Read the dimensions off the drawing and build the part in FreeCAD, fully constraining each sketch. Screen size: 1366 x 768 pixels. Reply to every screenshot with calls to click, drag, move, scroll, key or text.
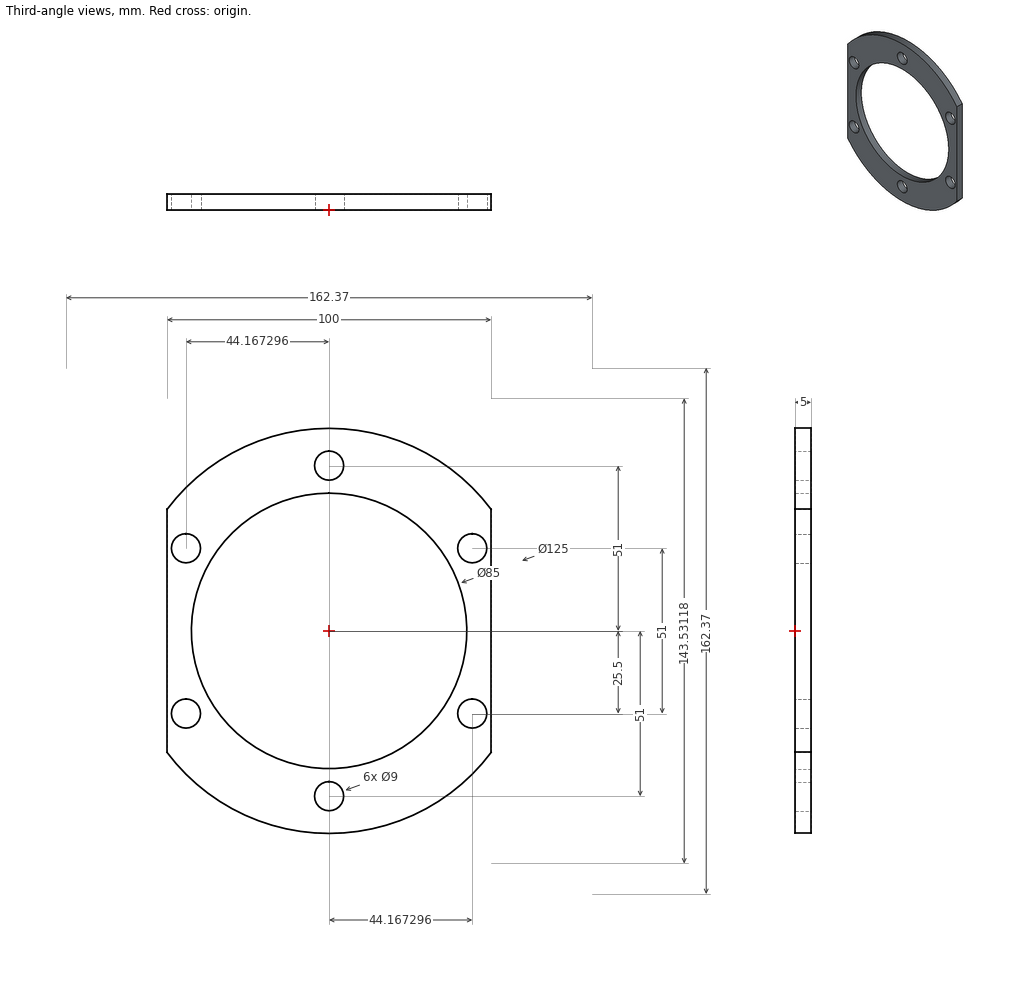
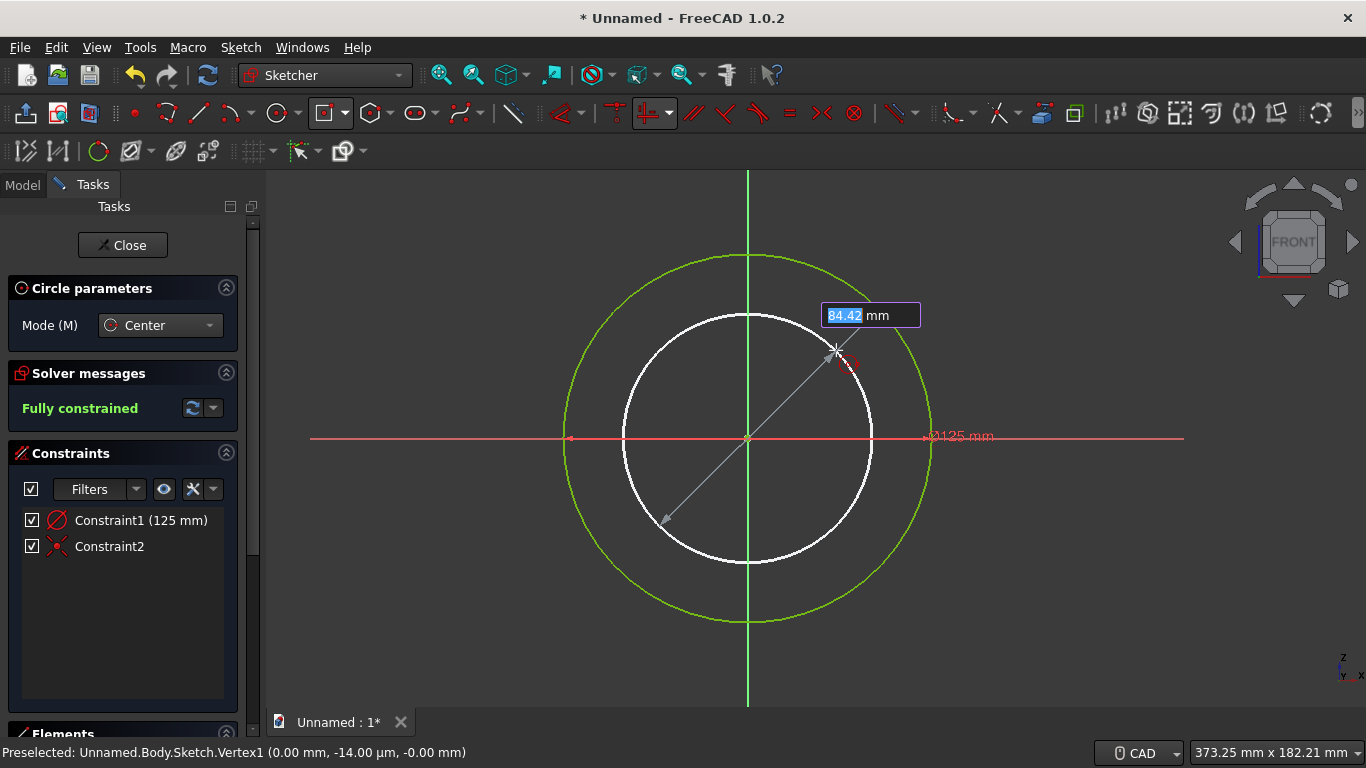
text(85)
key(Return)
key(Escape)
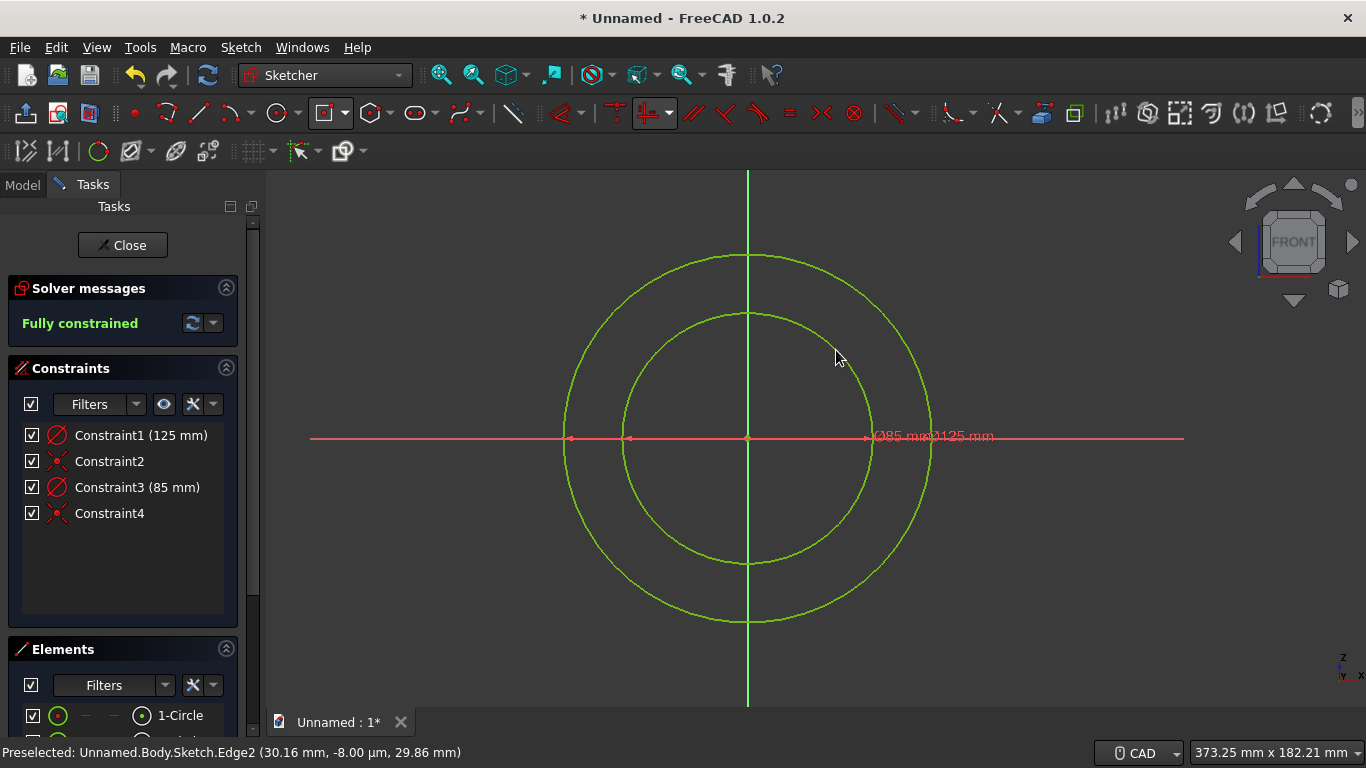
click(123, 245)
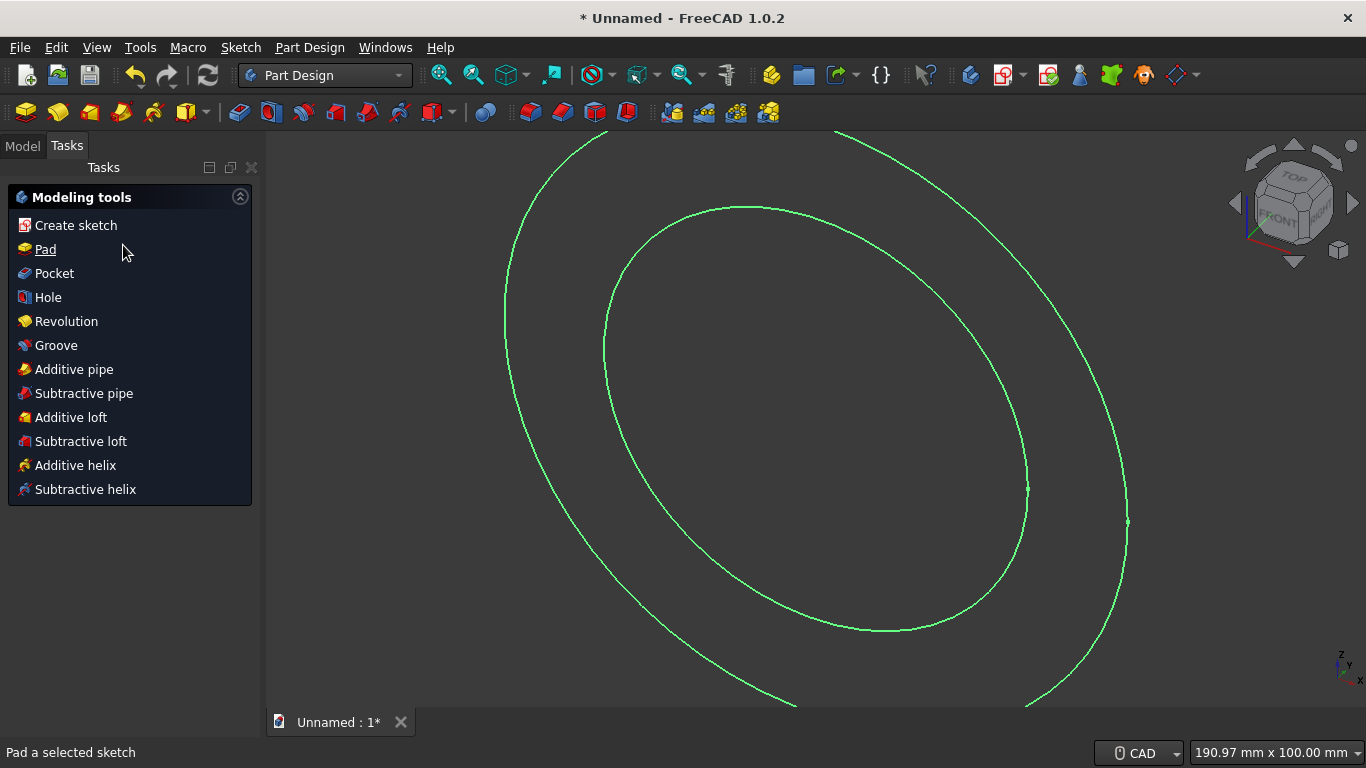
click(26, 112)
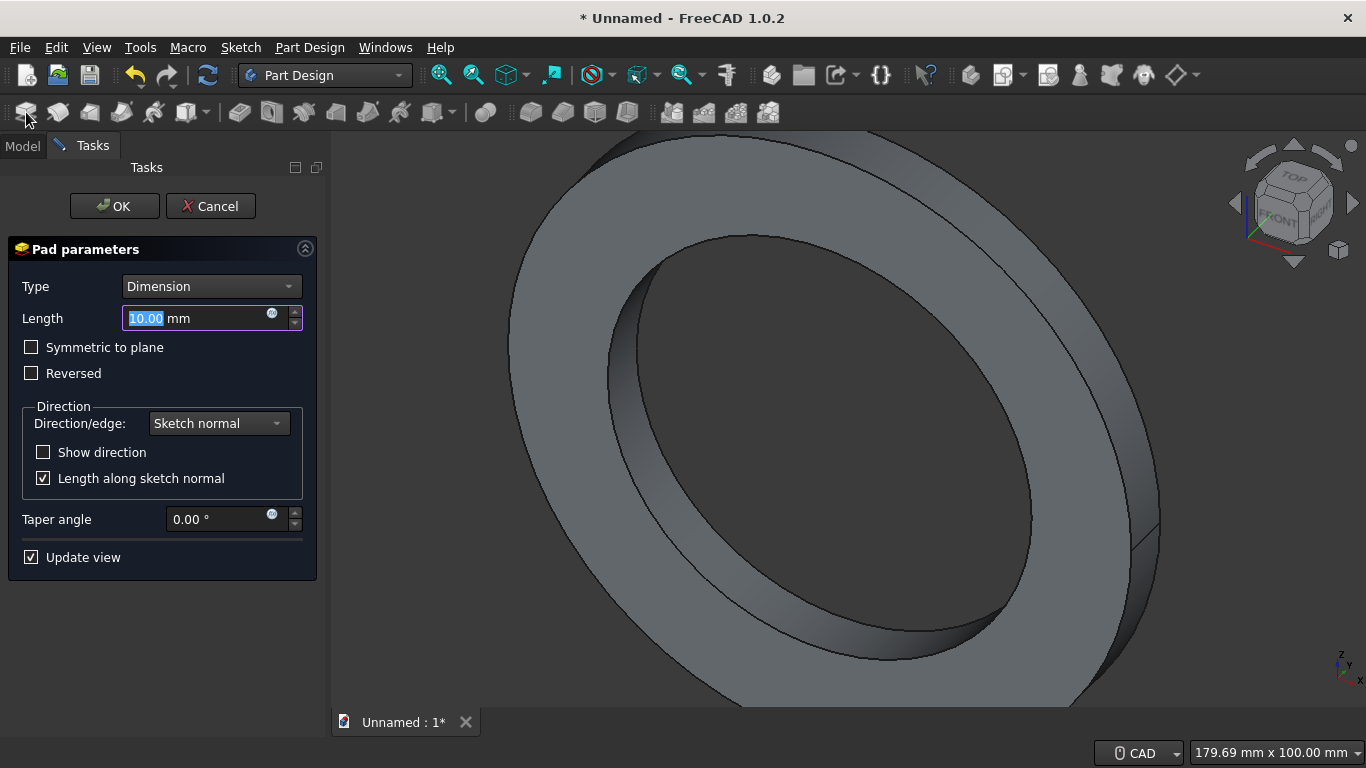
text(5)
key(Tab)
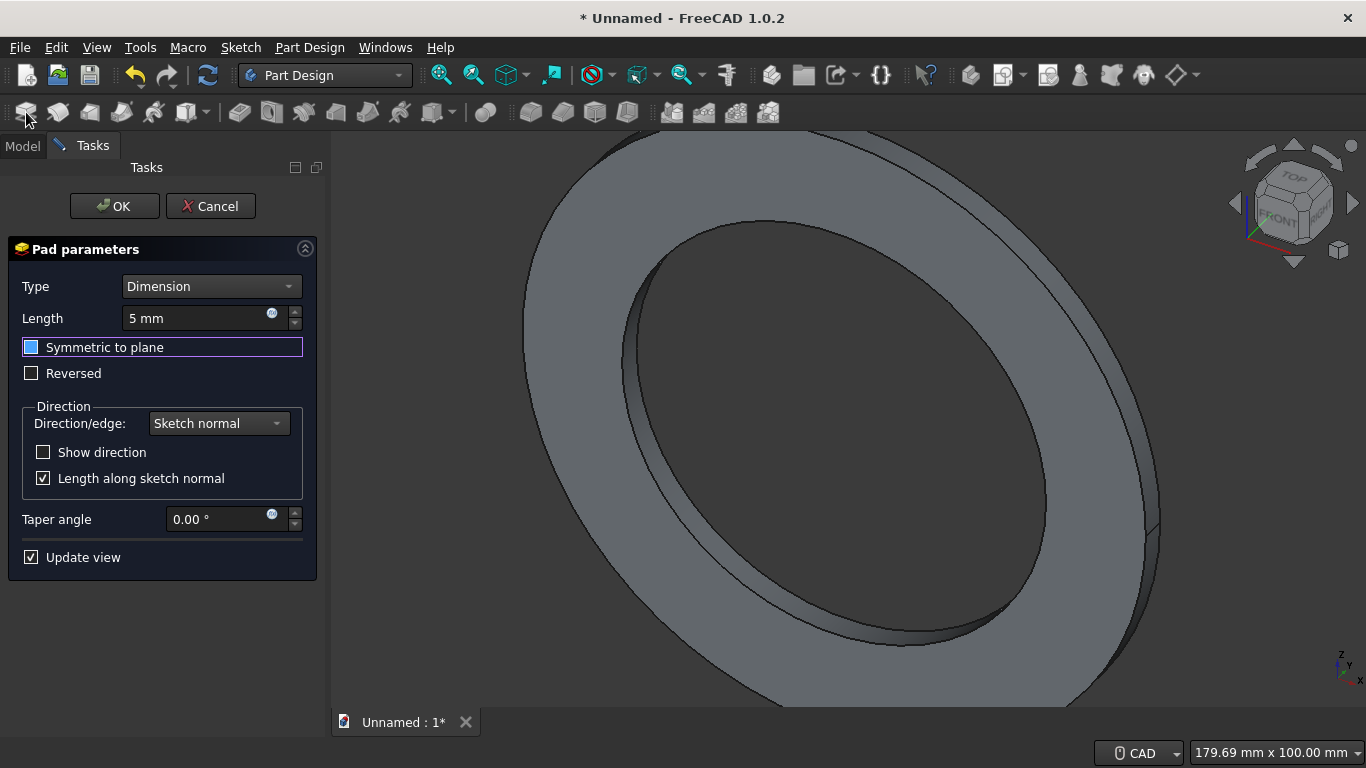
click(30, 373)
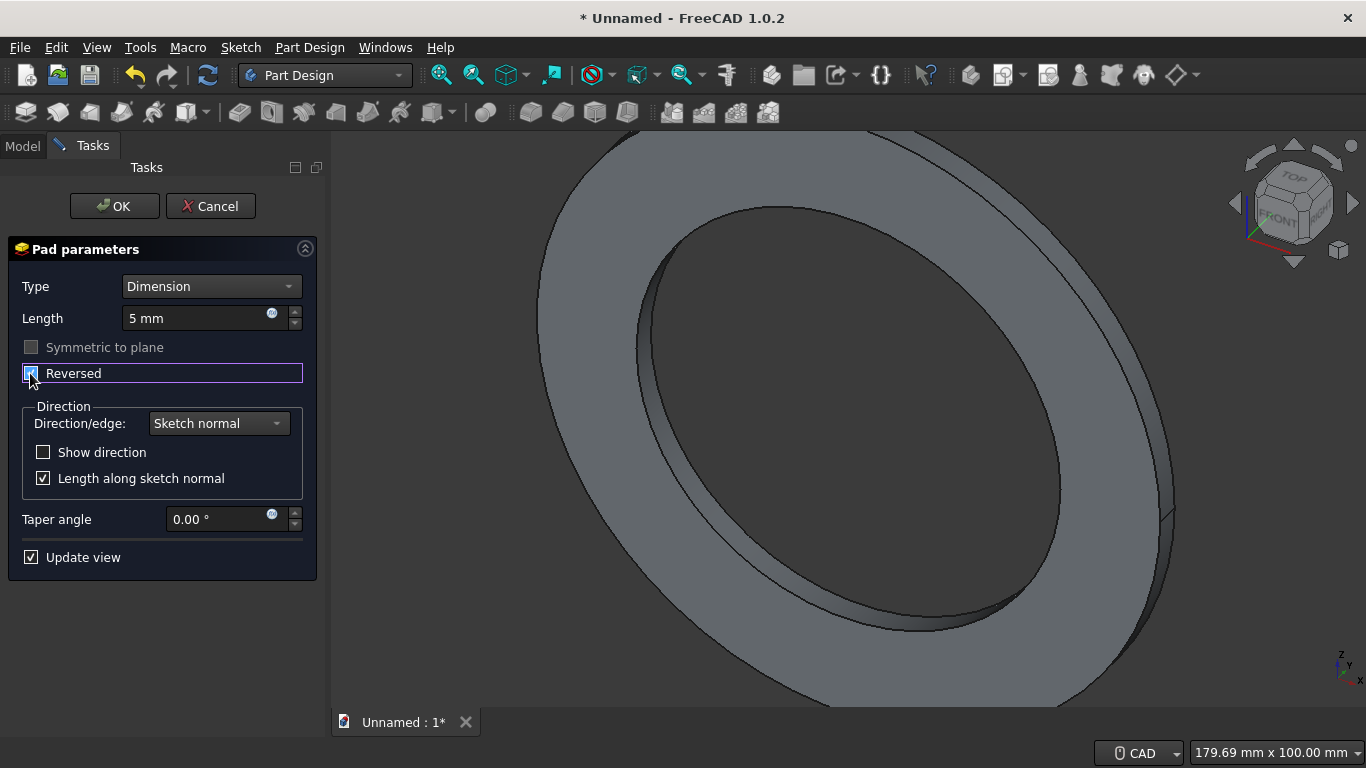
click(115, 206)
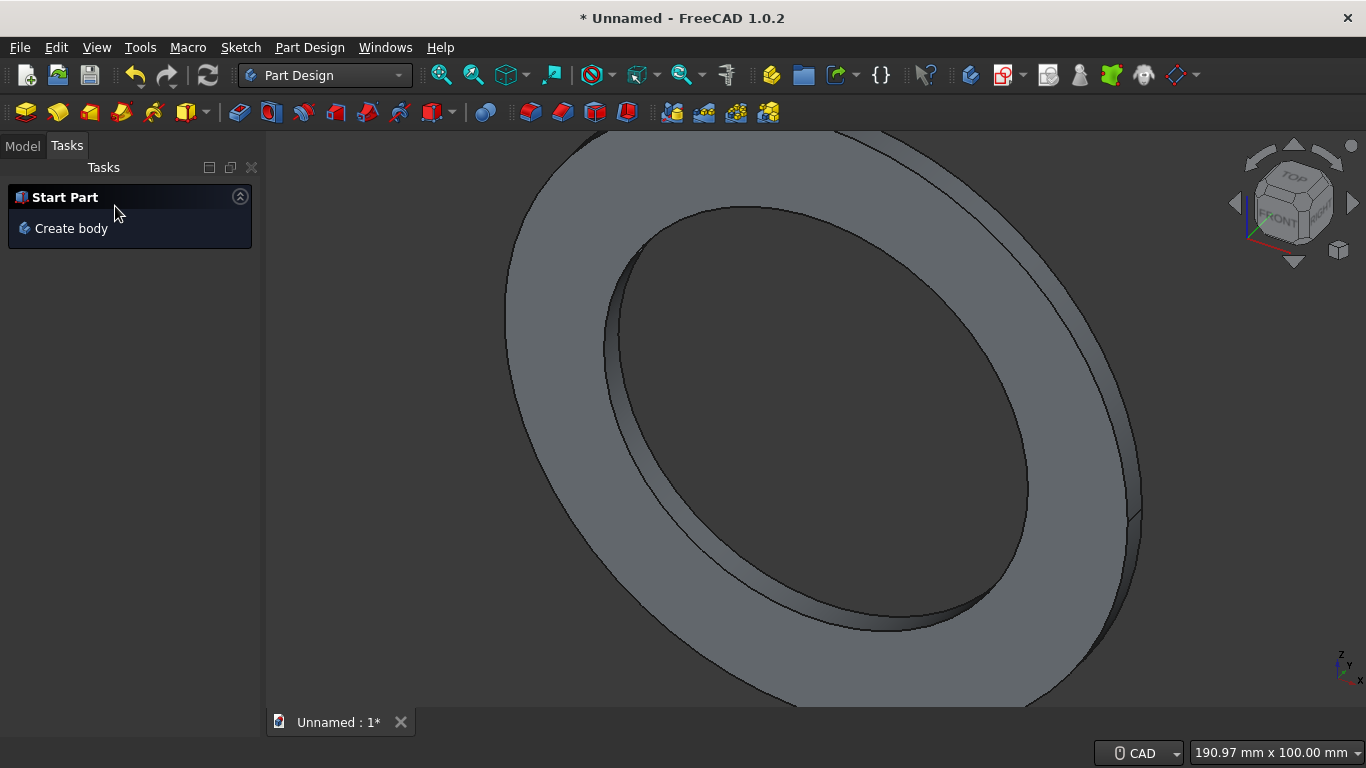
click(442, 76)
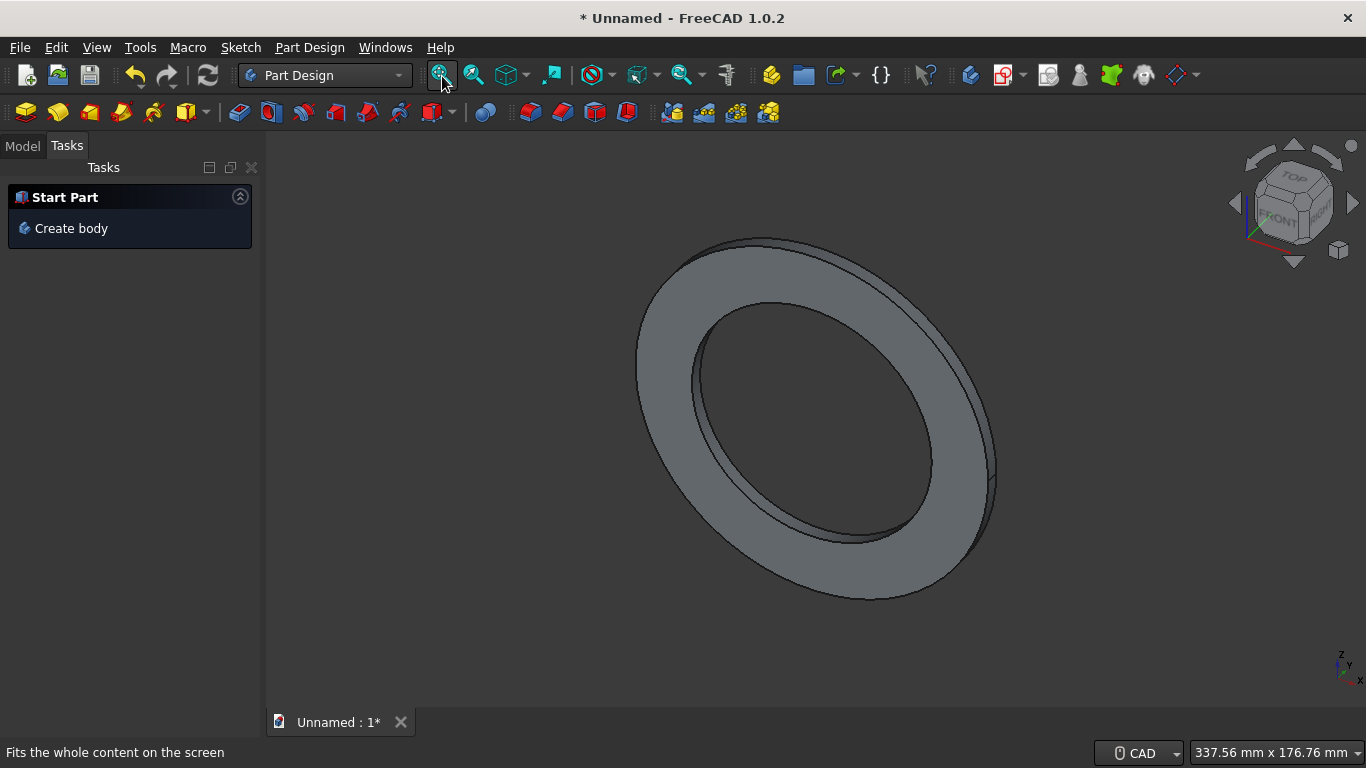
key(4)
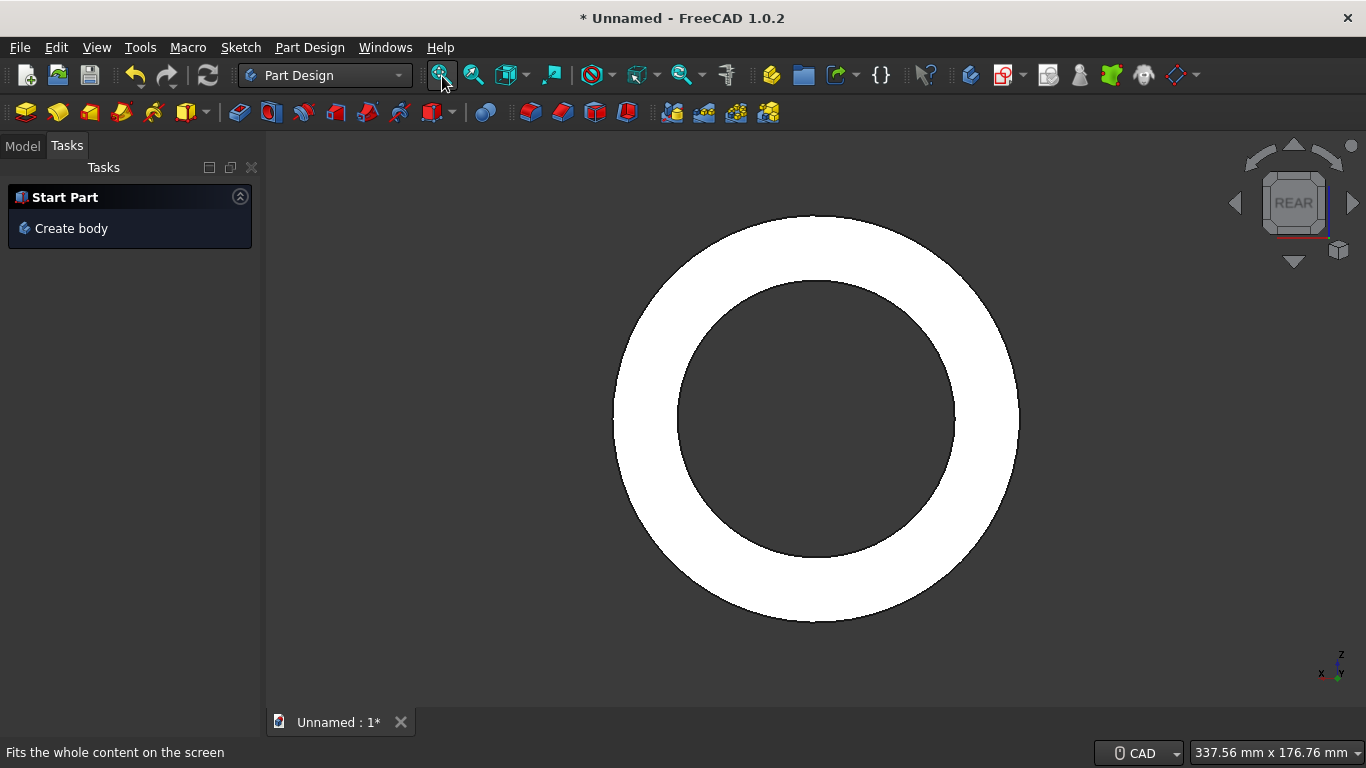
click(642, 418)